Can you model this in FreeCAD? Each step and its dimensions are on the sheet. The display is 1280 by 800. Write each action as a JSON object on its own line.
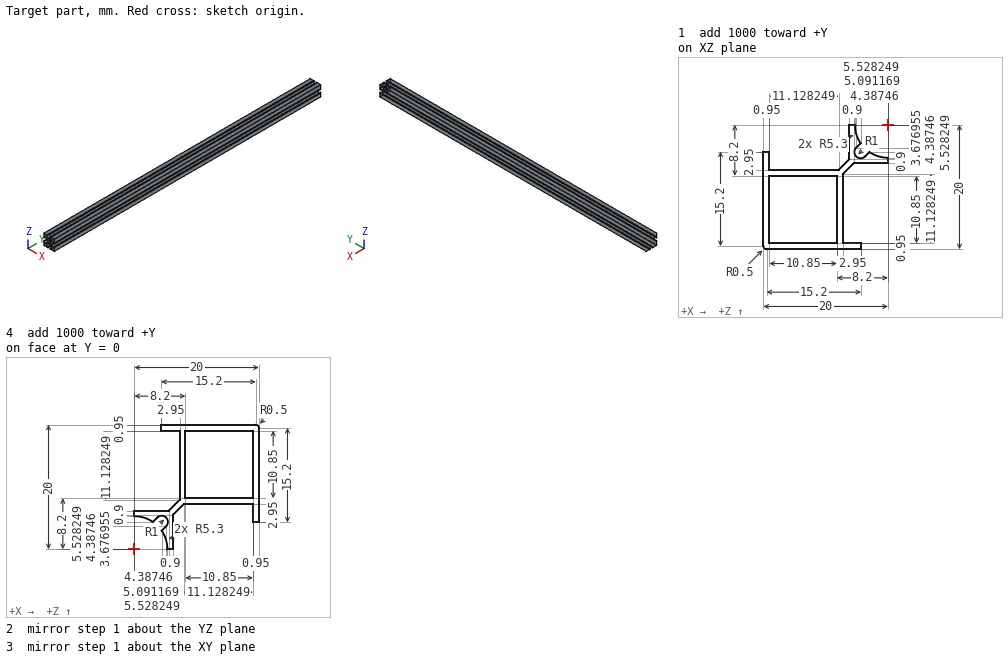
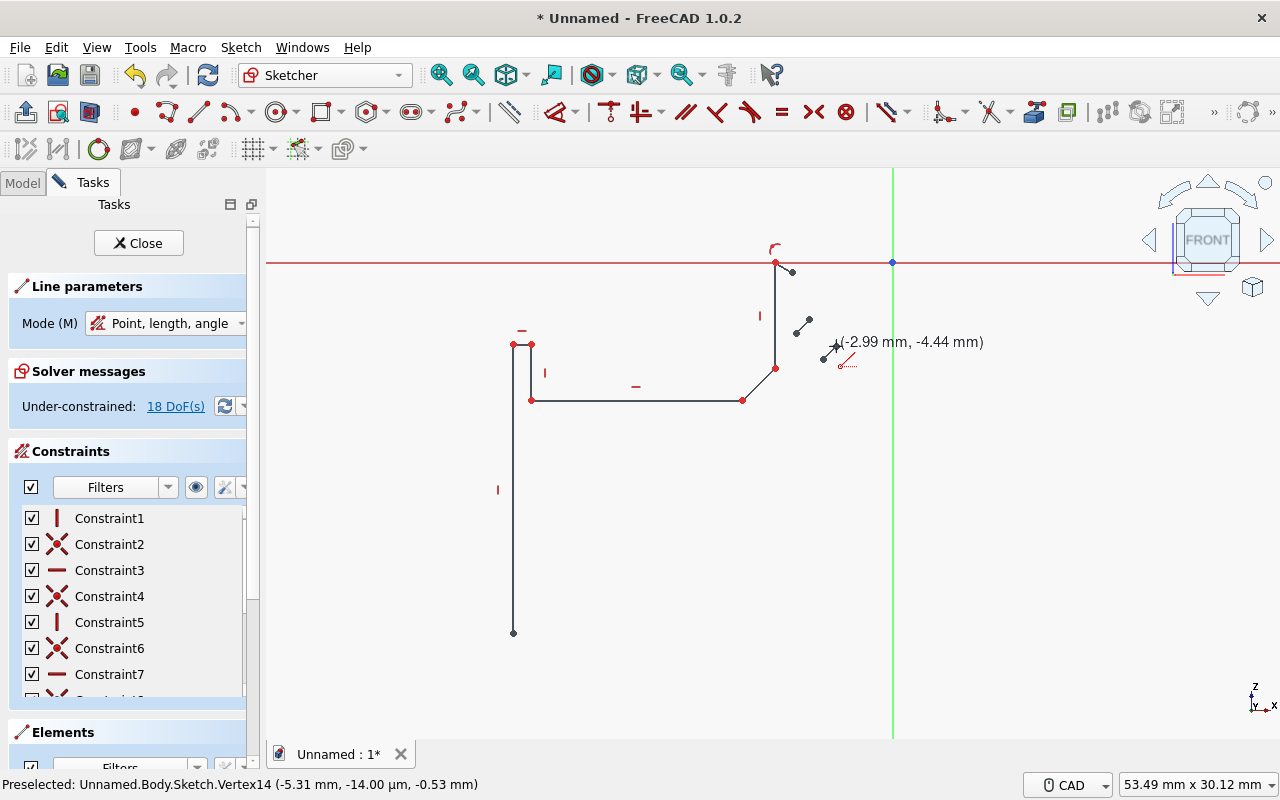
{"action": "left_click", "coordinate": [168, 112]}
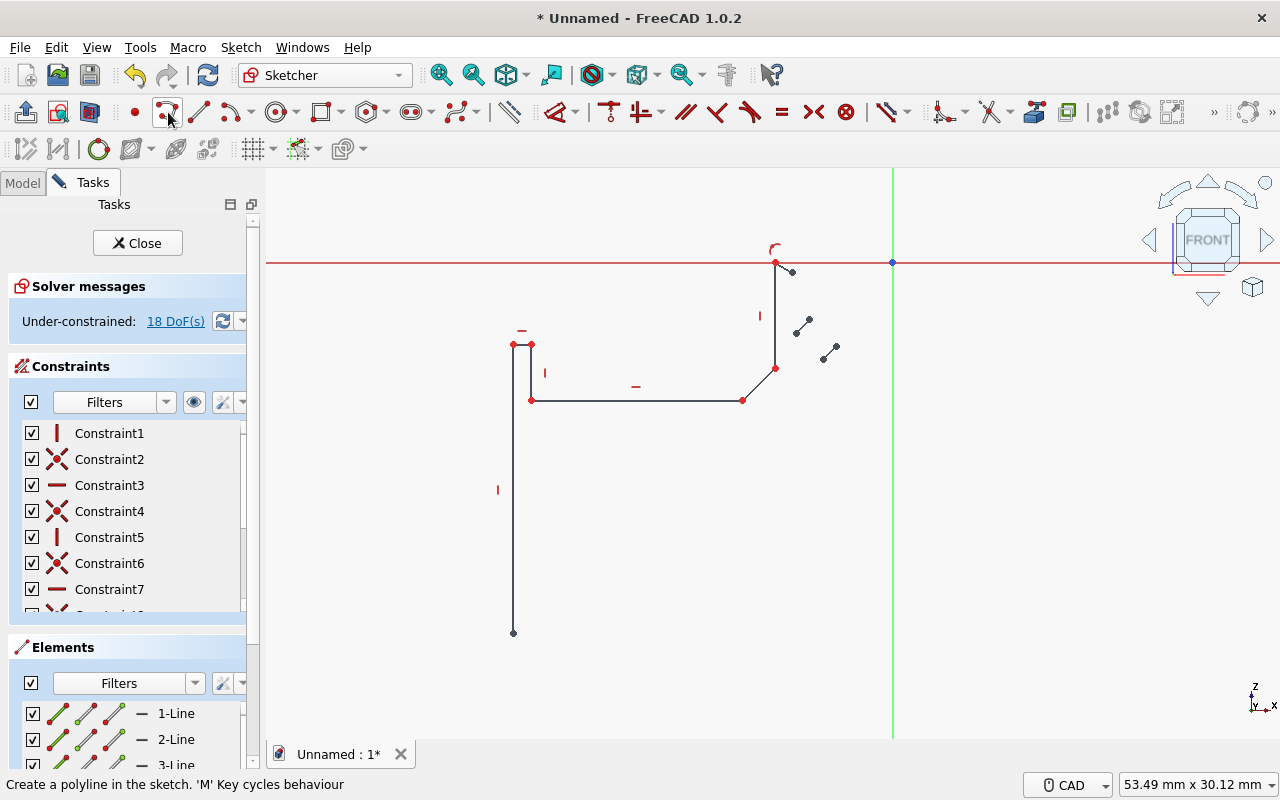
{"action": "left_click", "coordinate": [893, 363]}
{"action": "left_click", "coordinate": [884, 380]}
{"action": "left_click", "coordinate": [788, 380]}
{"action": "left_click", "coordinate": [755, 413]}
{"action": "left_click", "coordinate": [755, 624]}
{"action": "left_click", "coordinate": [811, 624]}
{"action": "left_click", "coordinate": [811, 642]}
{"action": "left_click", "coordinate": [523, 642]}
{"action": "right_click", "coordinate": [523, 642]}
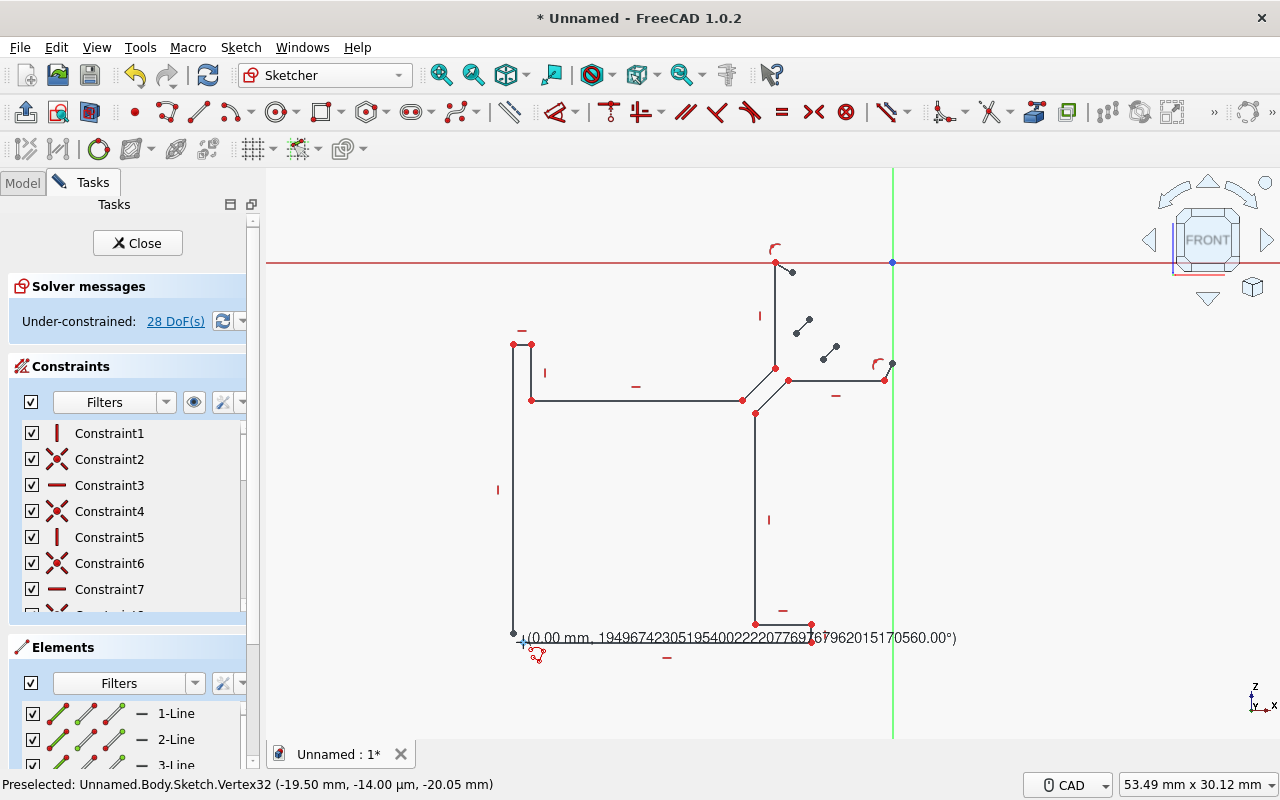
{"action": "left_click", "coordinate": [254, 112]}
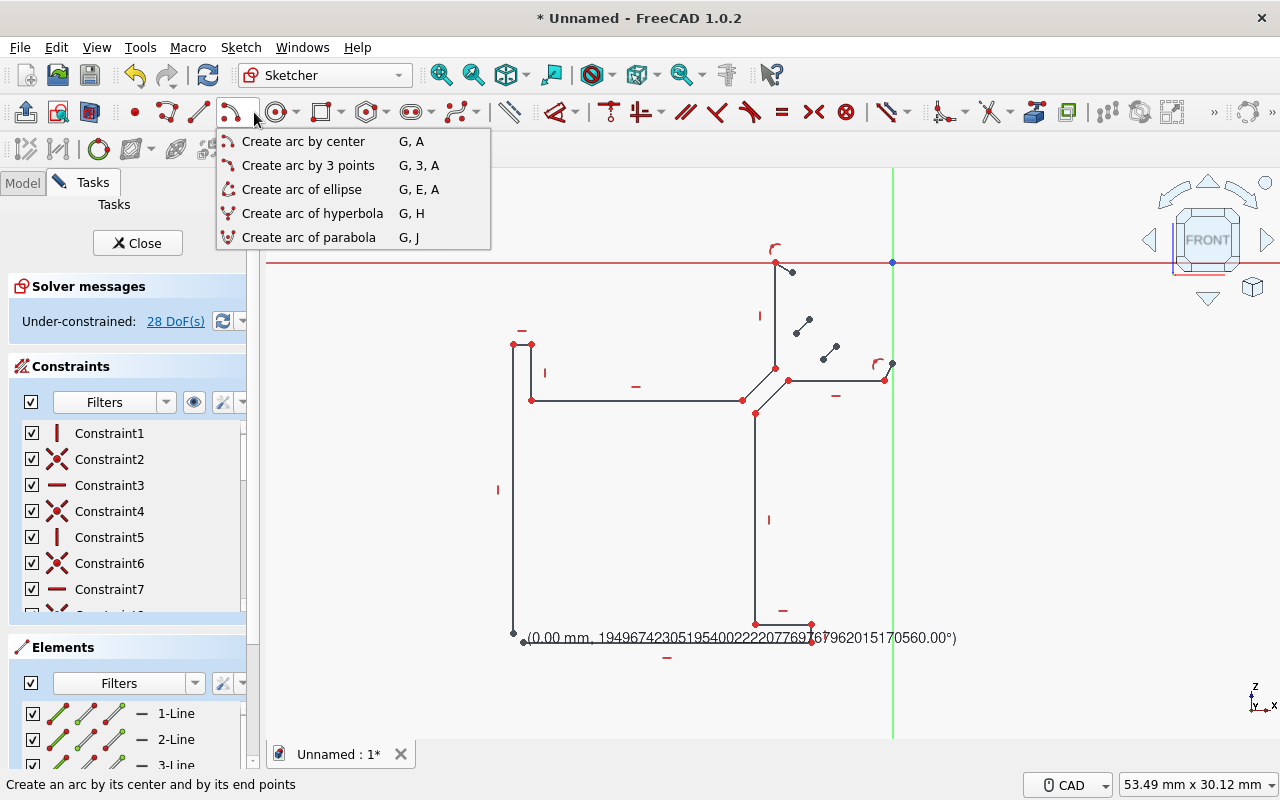
{"action": "left_click", "coordinate": [354, 165]}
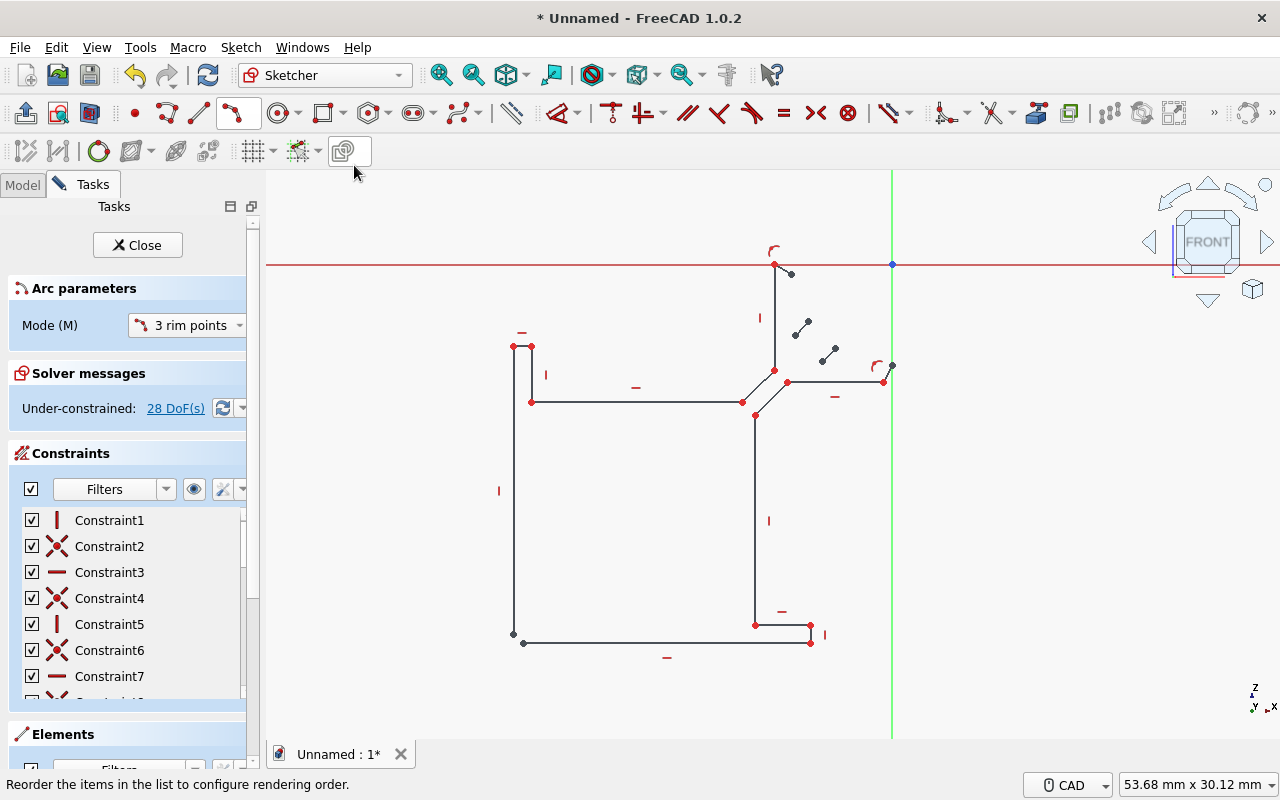
{"action": "scroll", "coordinate": [792, 265], "scroll_direction": "up", "scroll_amount": 4}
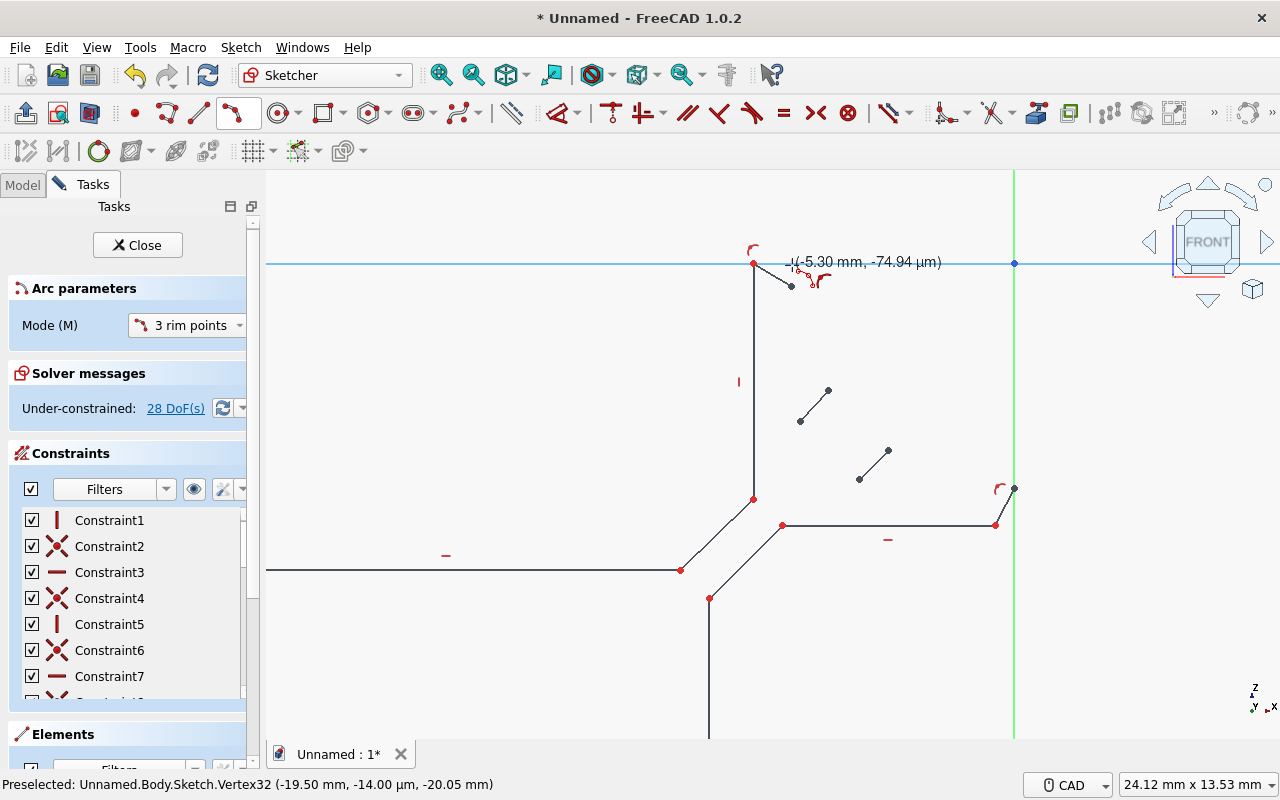
{"action": "left_click", "coordinate": [791, 286]}
{"action": "left_click", "coordinate": [829, 390]}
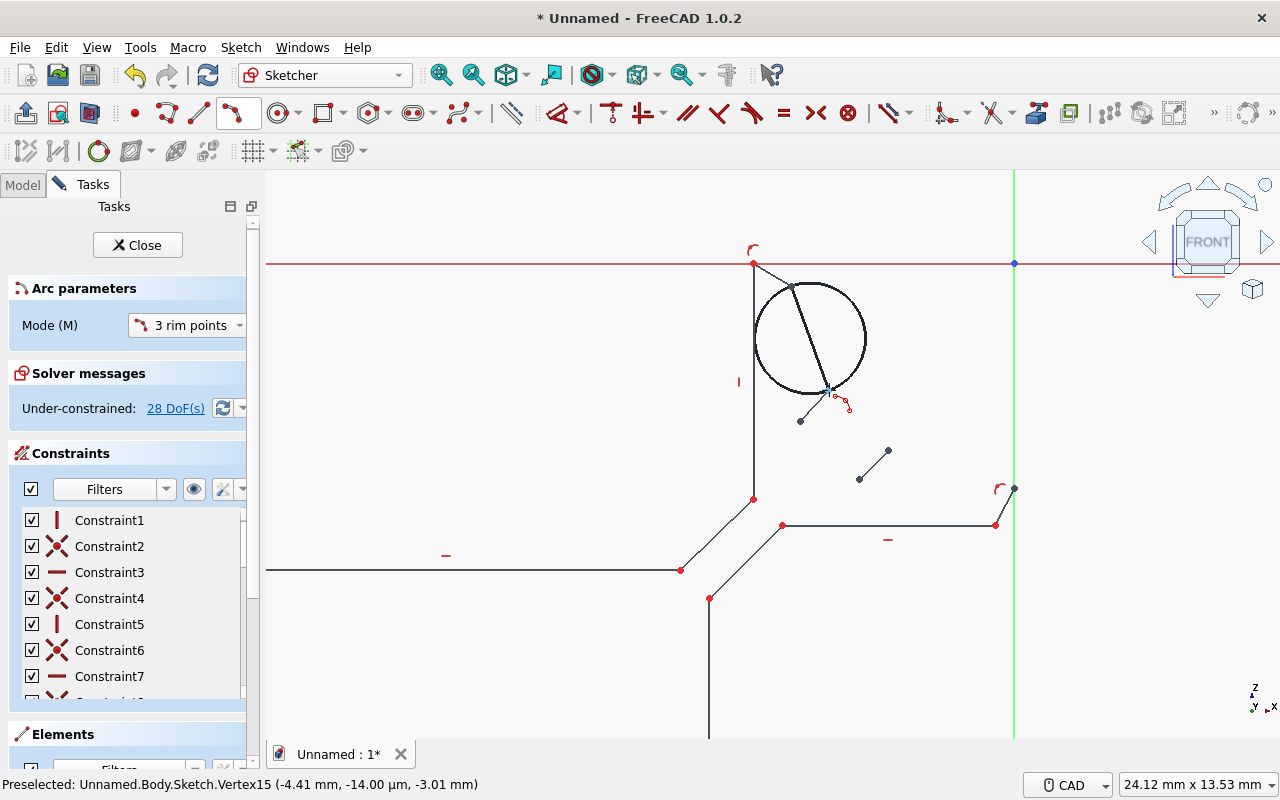
{"action": "scroll", "coordinate": [801, 329], "scroll_direction": "up", "scroll_amount": 3}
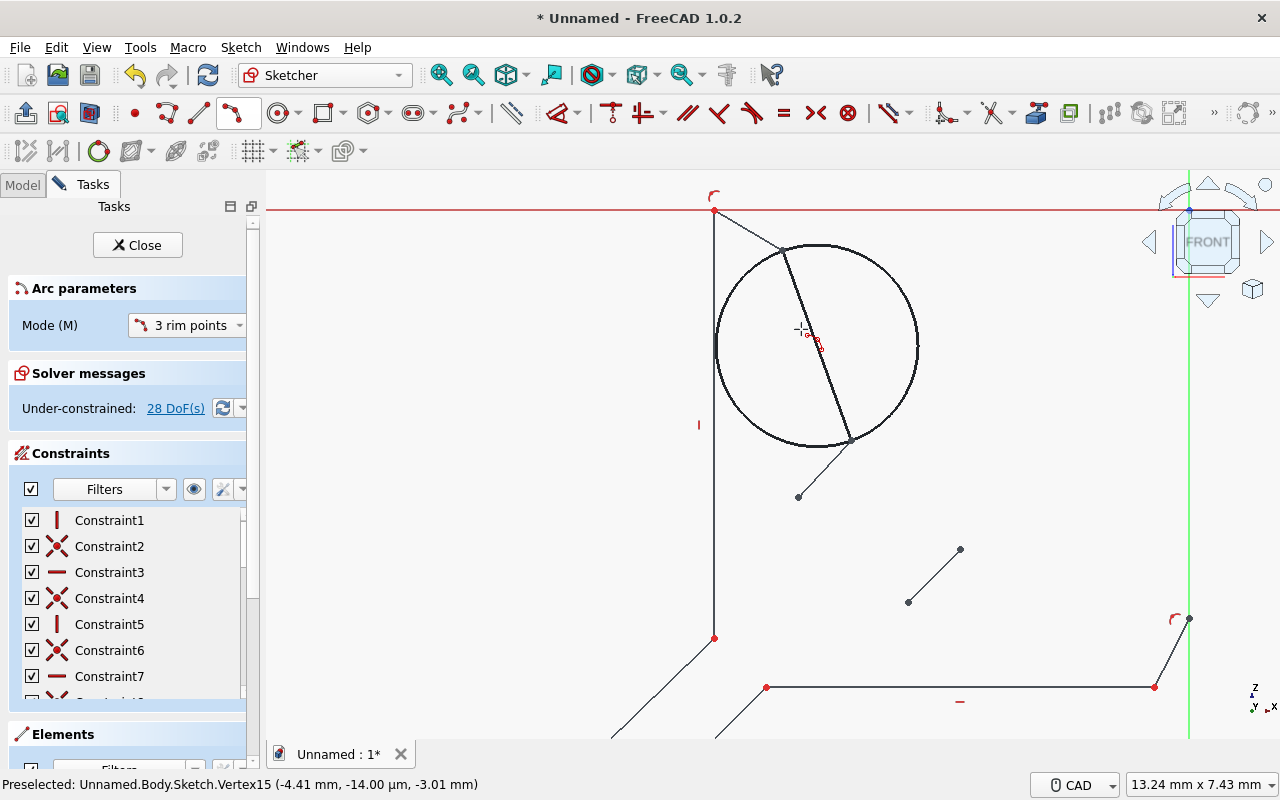
{"action": "left_click", "coordinate": [801, 329]}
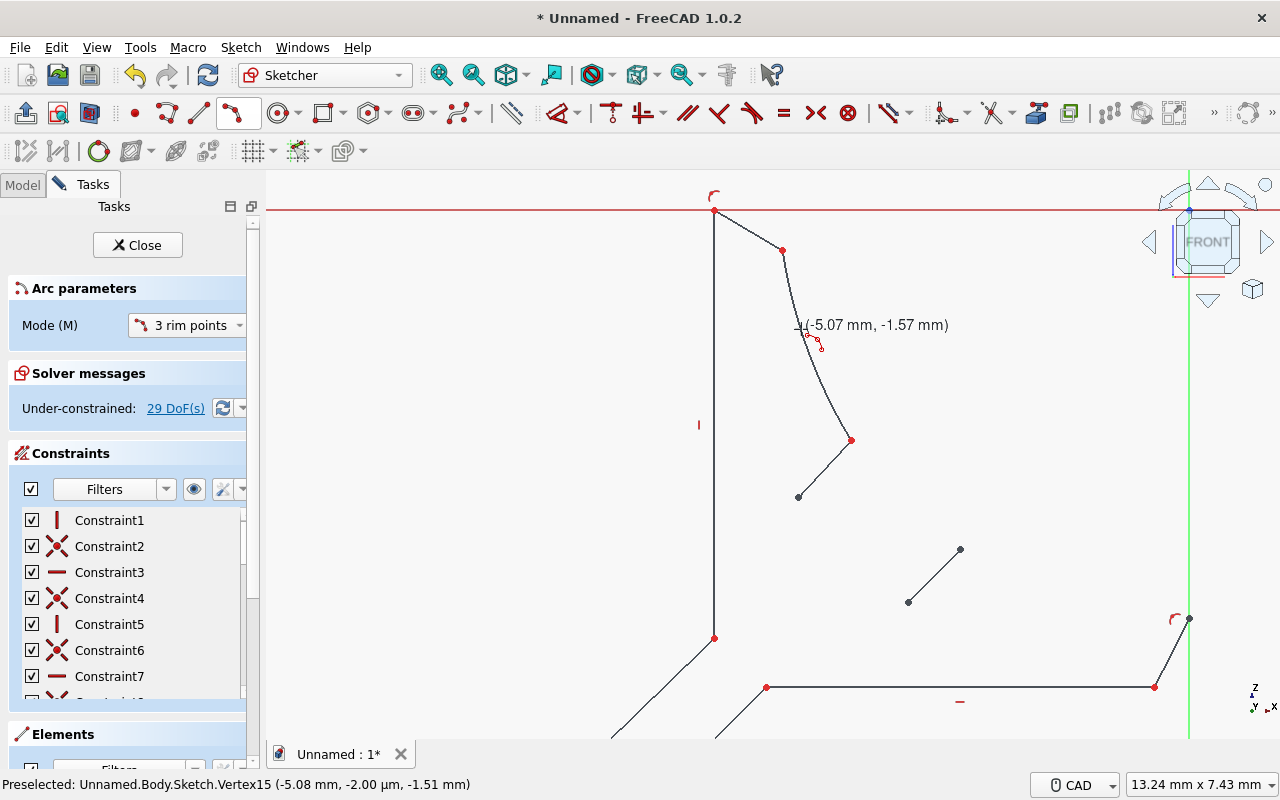
{"action": "left_click", "coordinate": [799, 497]}
{"action": "left_click", "coordinate": [908, 602]}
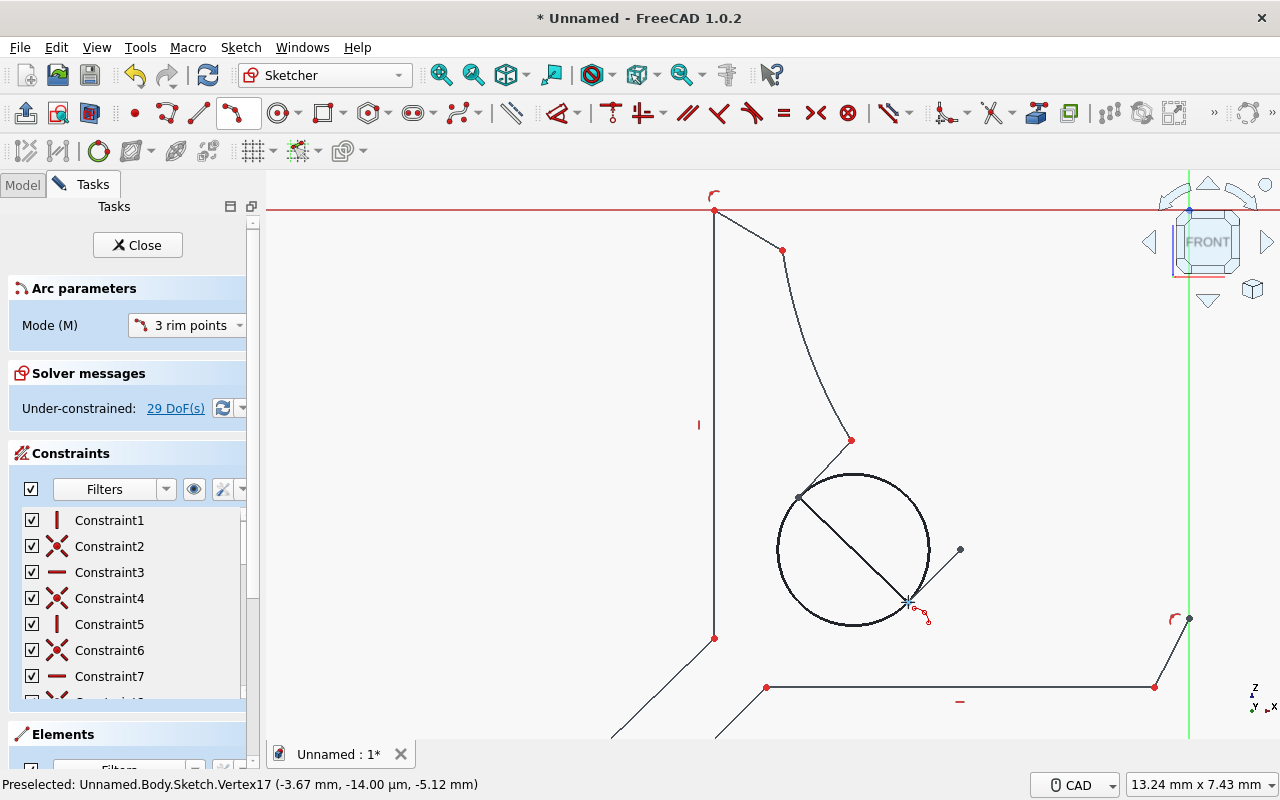
{"action": "scroll", "coordinate": [797, 284], "scroll_direction": "down", "scroll_amount": 7}